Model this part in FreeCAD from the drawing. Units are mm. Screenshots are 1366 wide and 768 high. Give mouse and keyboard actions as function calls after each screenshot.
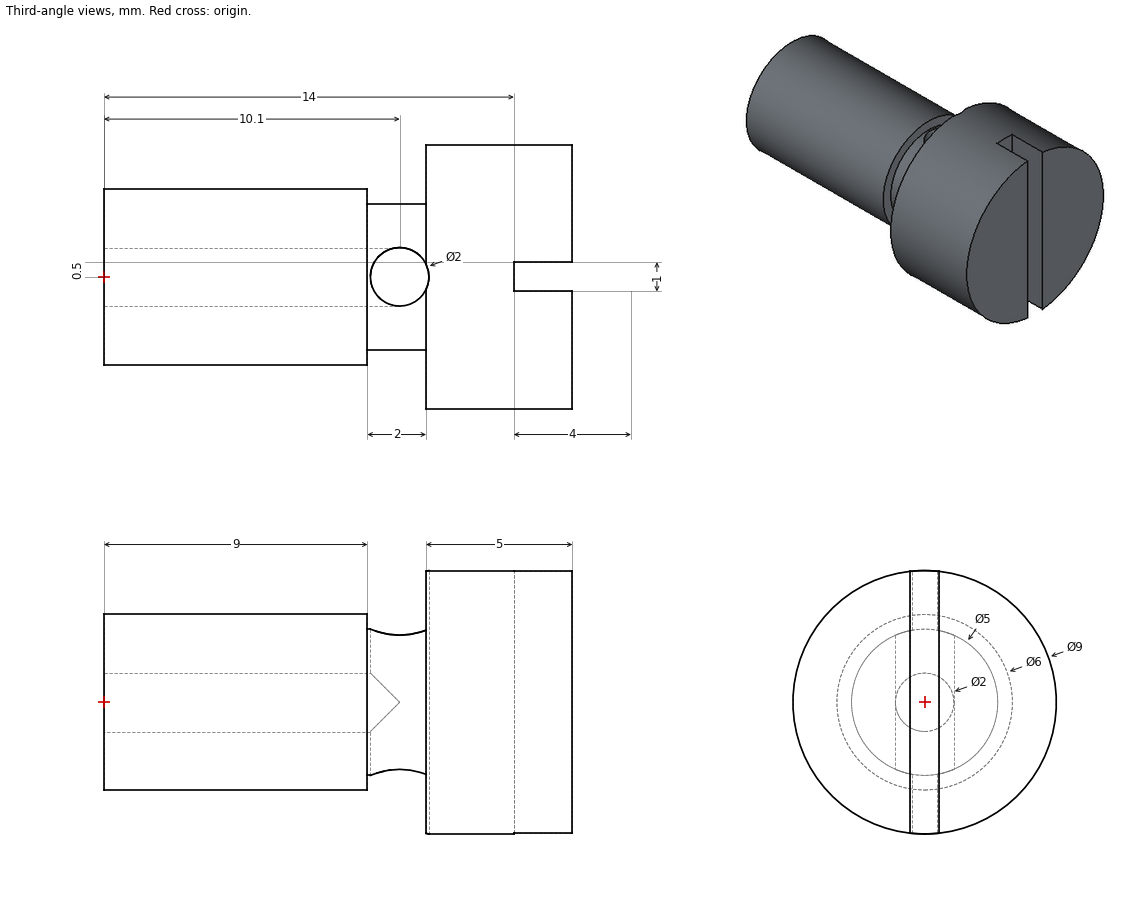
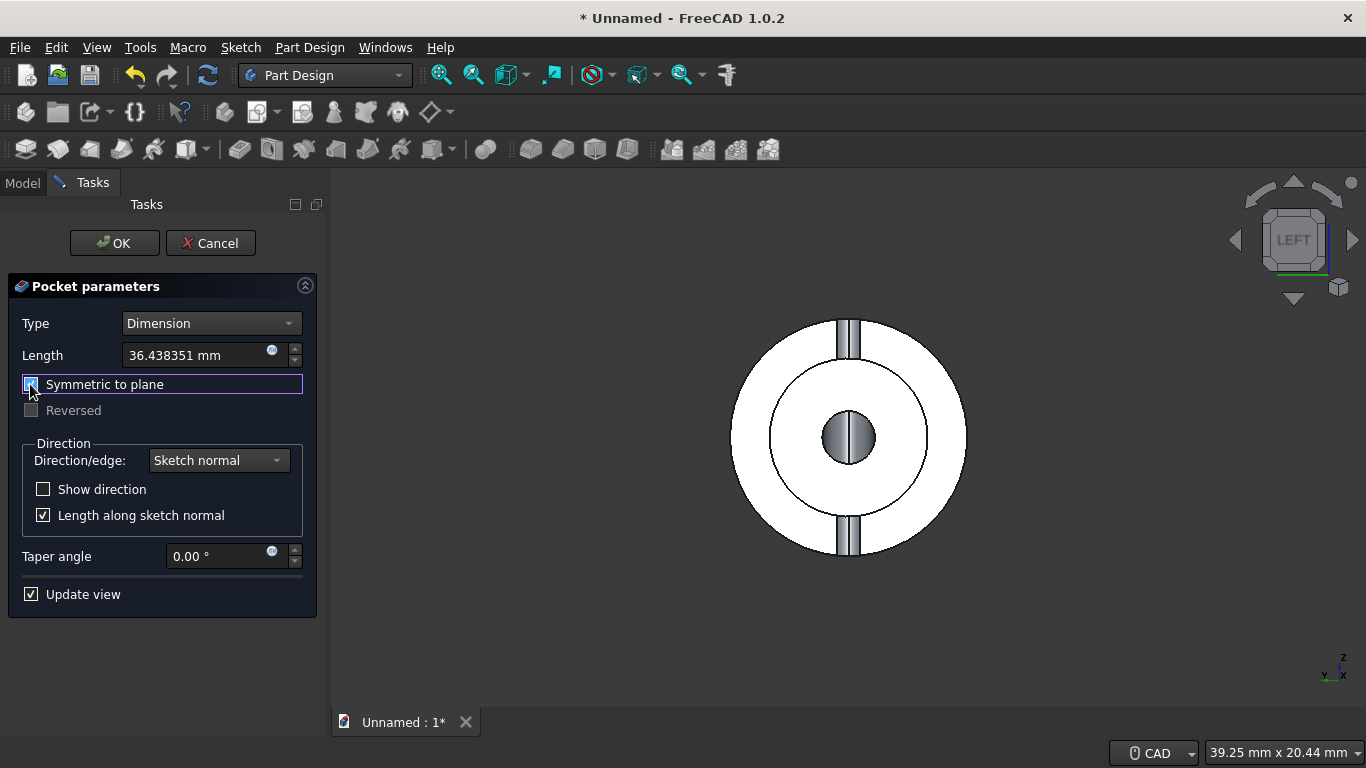
click(115, 243)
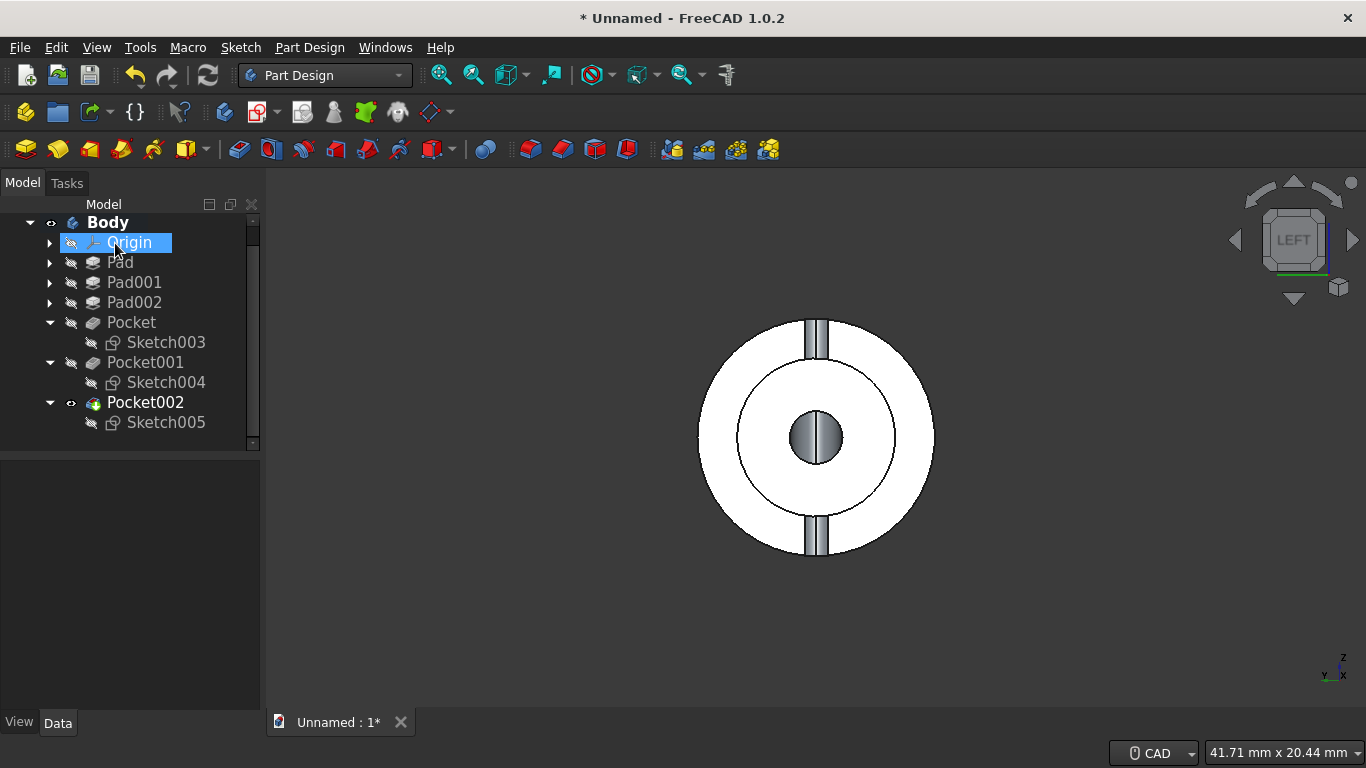
key(0)